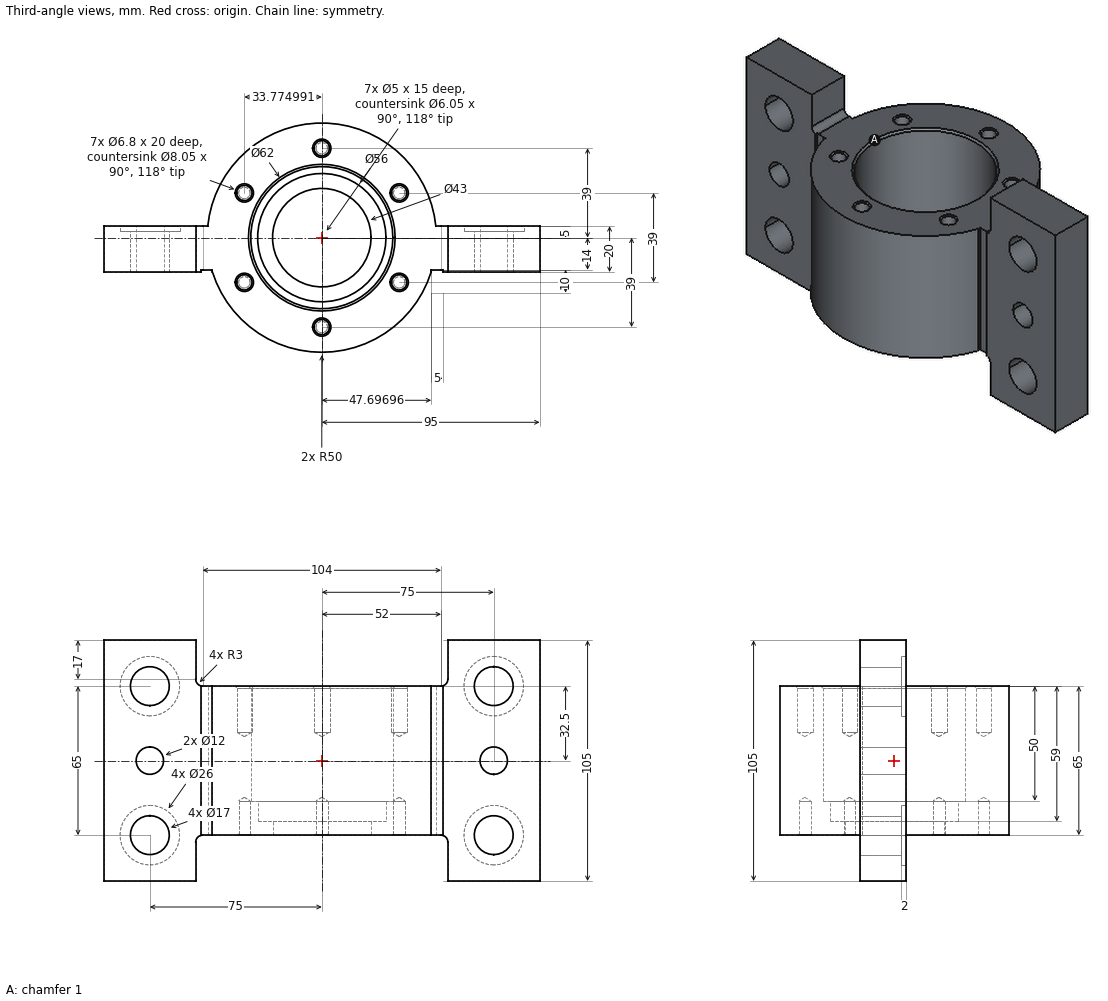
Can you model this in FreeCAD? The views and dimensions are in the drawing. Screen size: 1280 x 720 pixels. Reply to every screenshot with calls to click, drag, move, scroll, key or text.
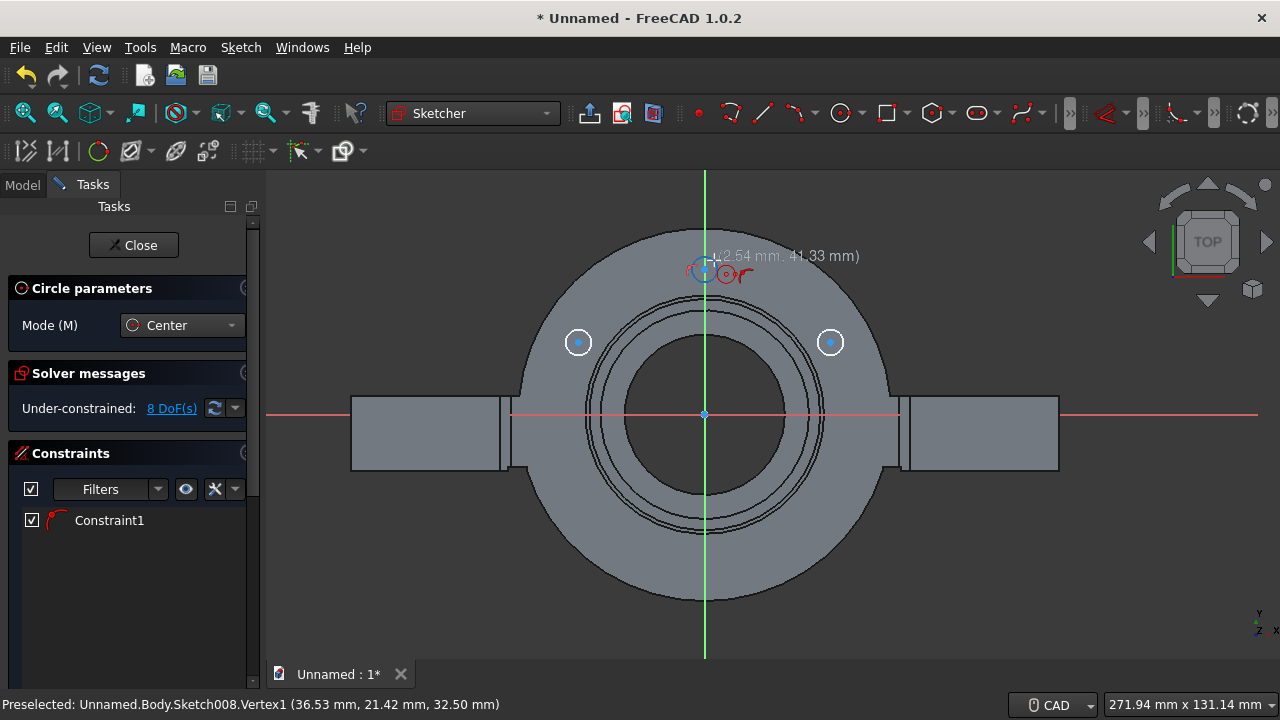
scroll(831, 487, up, 3)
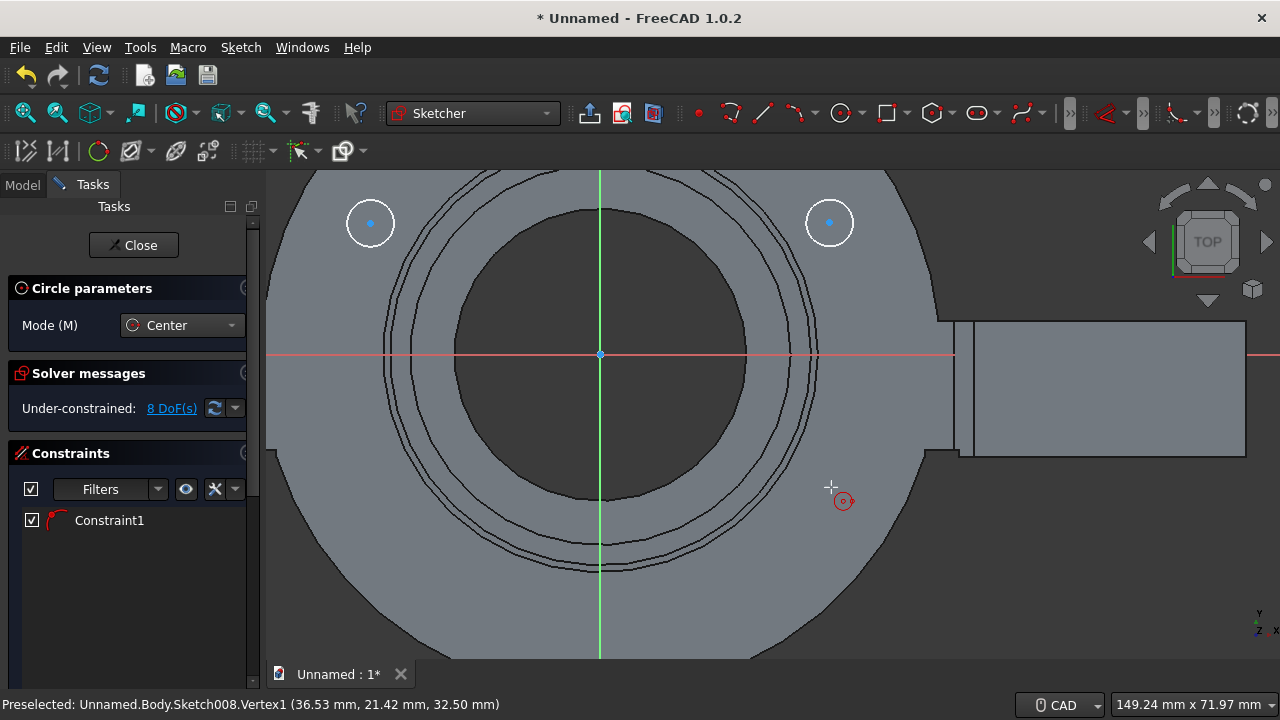
click(830, 487)
click(846, 471)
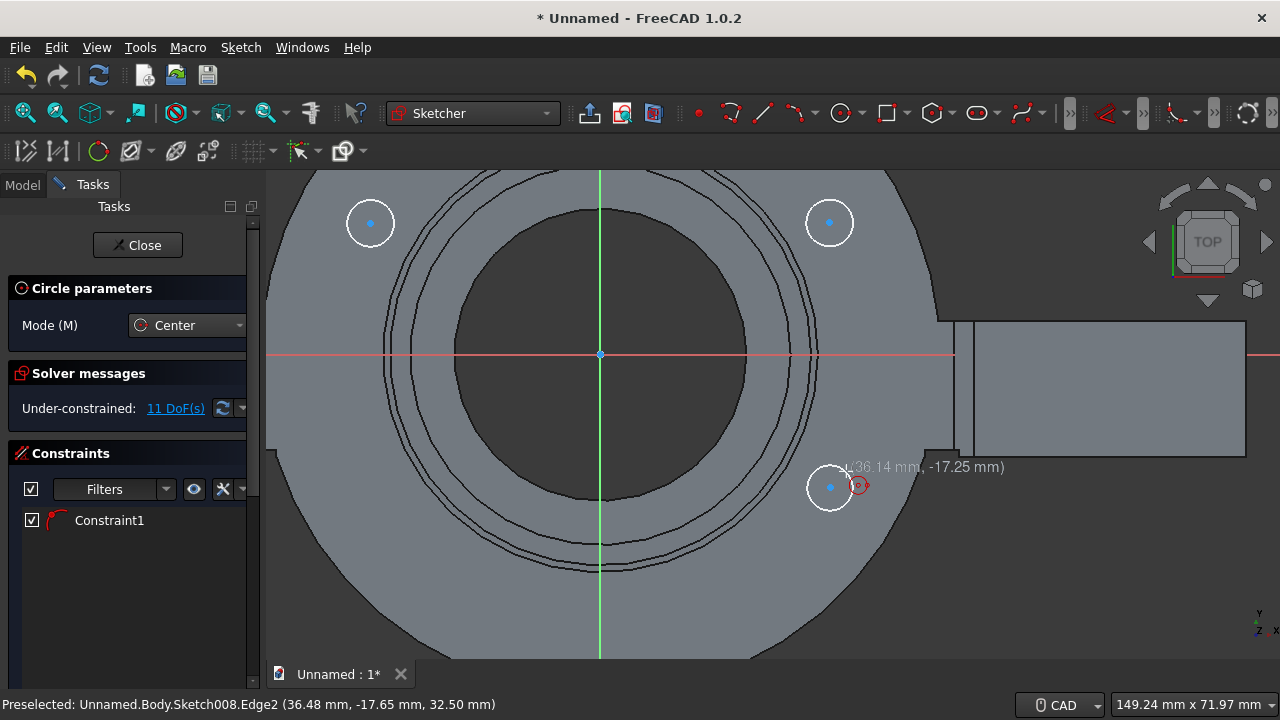
click(600, 620)
click(617, 603)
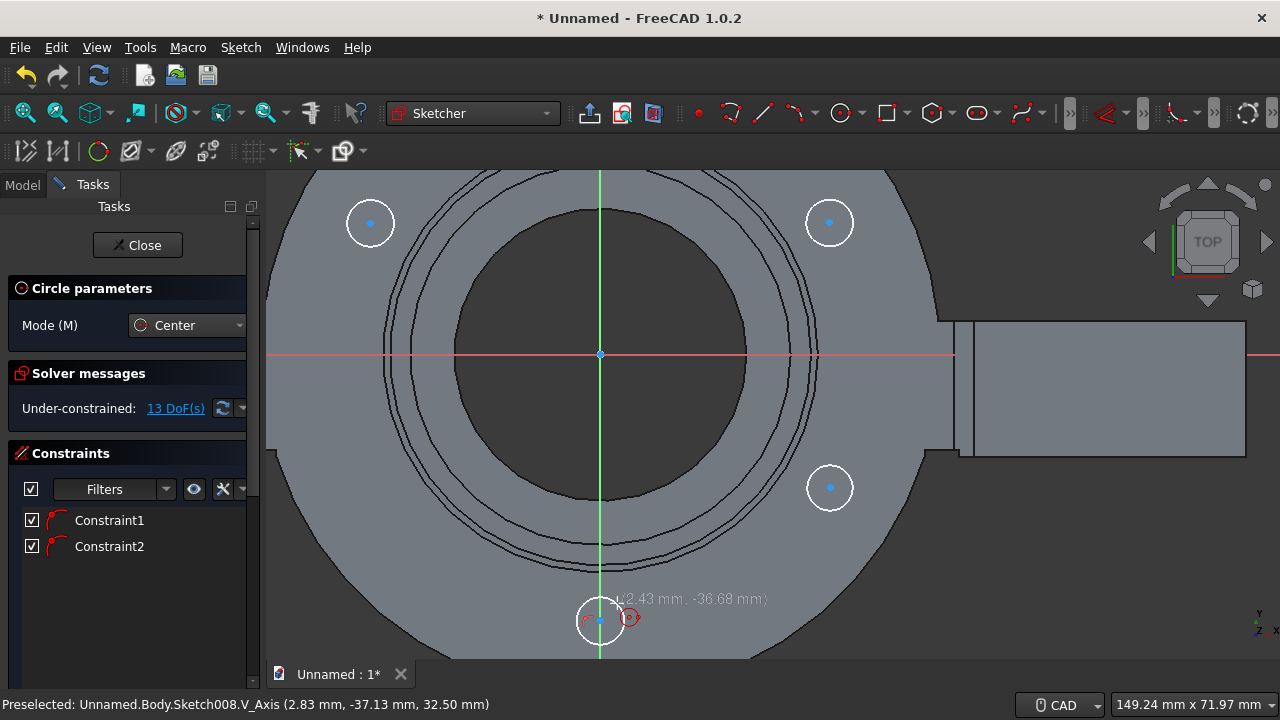
click(371, 487)
click(387, 471)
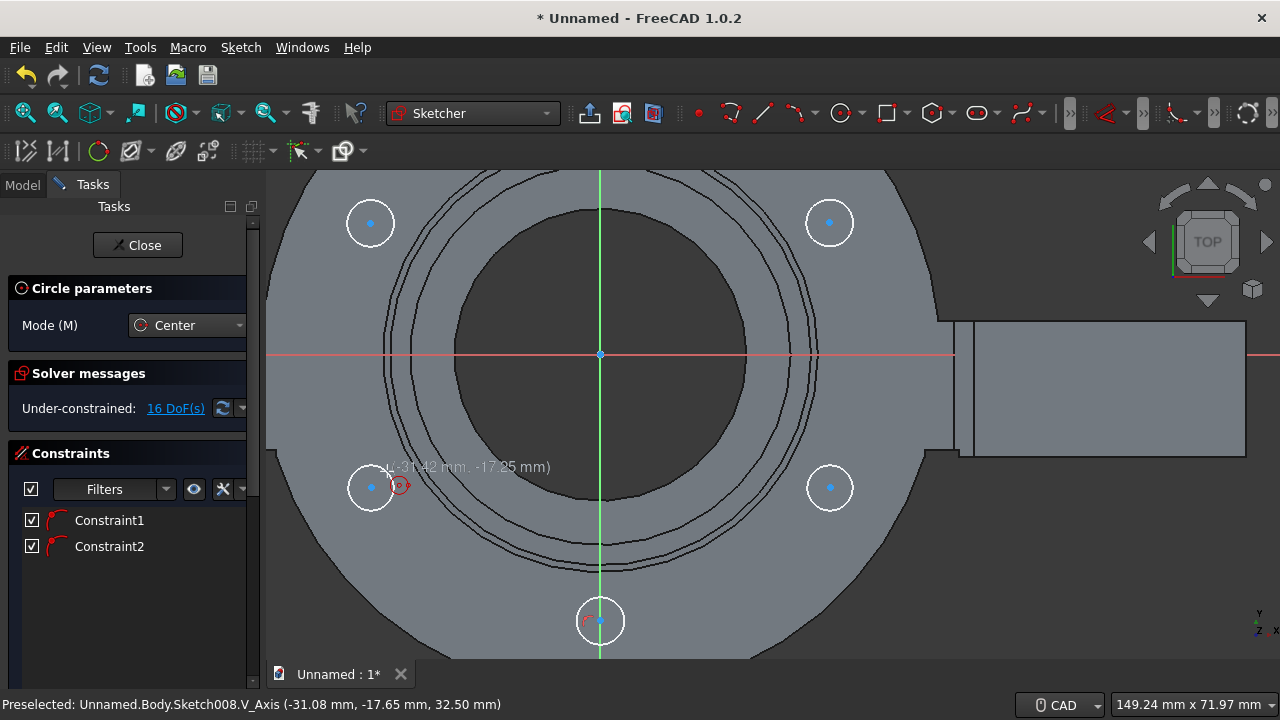
click(600, 355)
click(617, 338)
key(Escape)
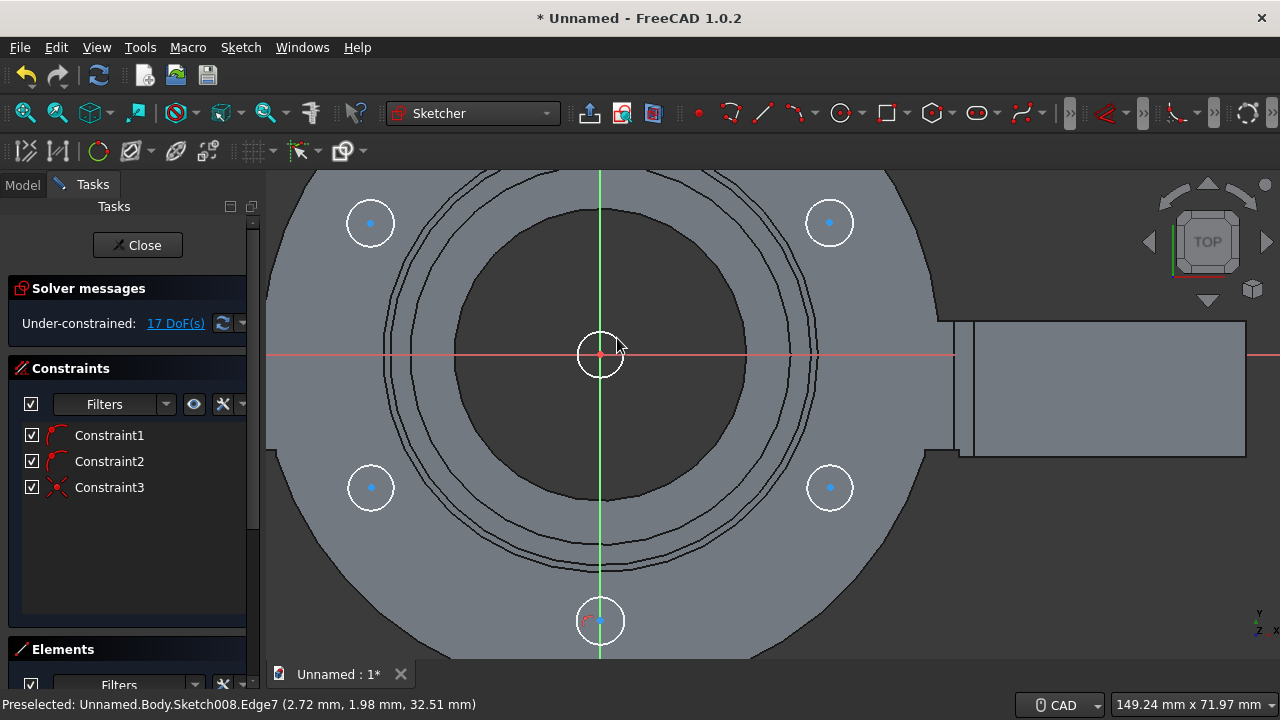
click(387, 207)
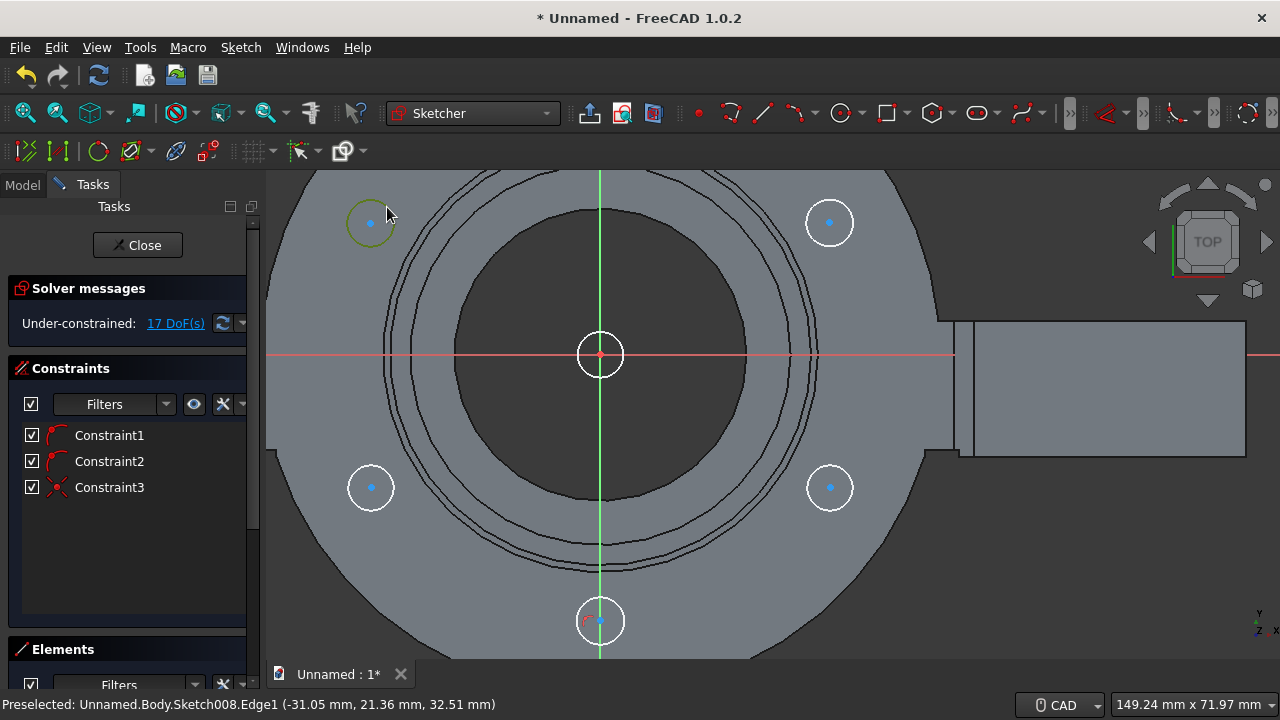
scroll(831, 487, down, 3)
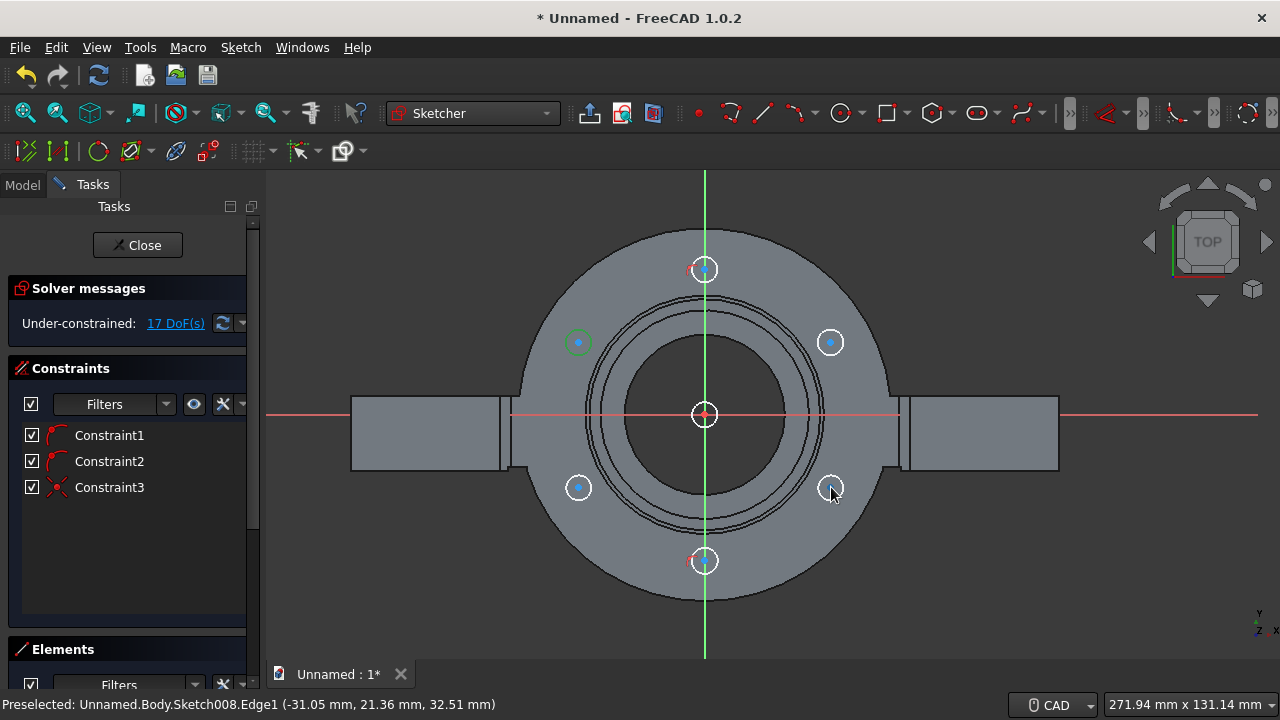
scroll(714, 261, up, 3)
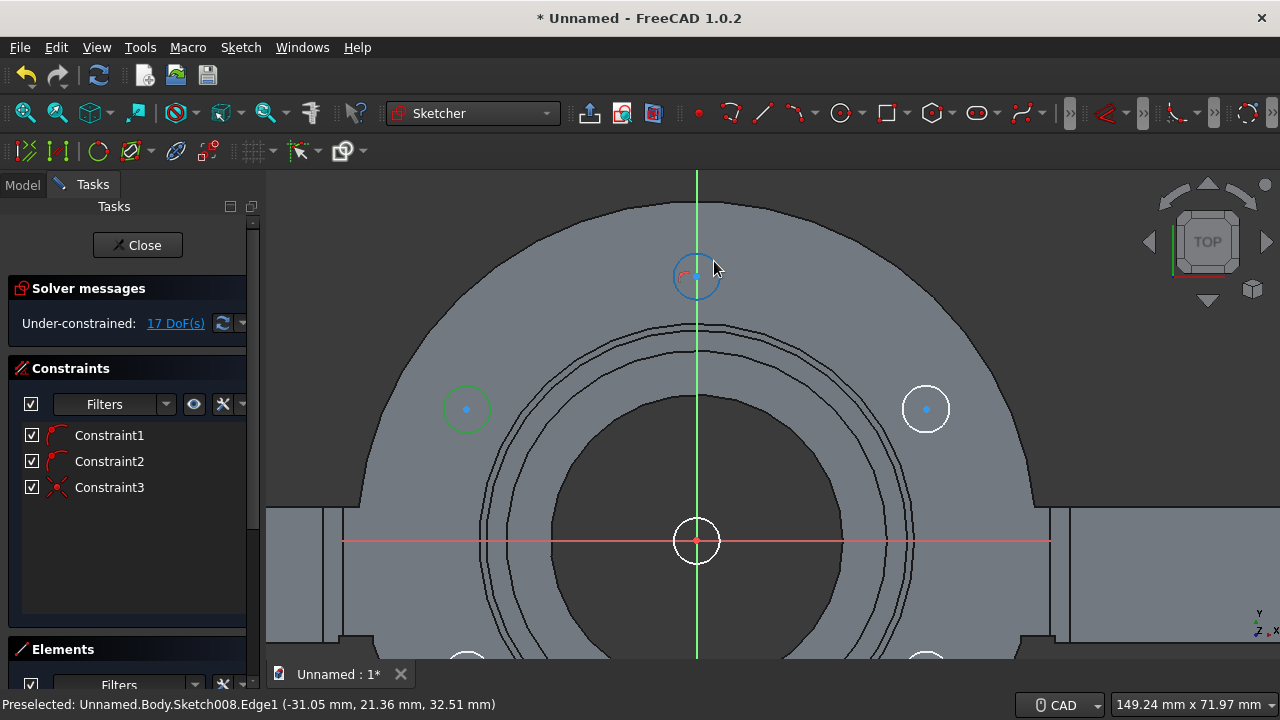
click(713, 260)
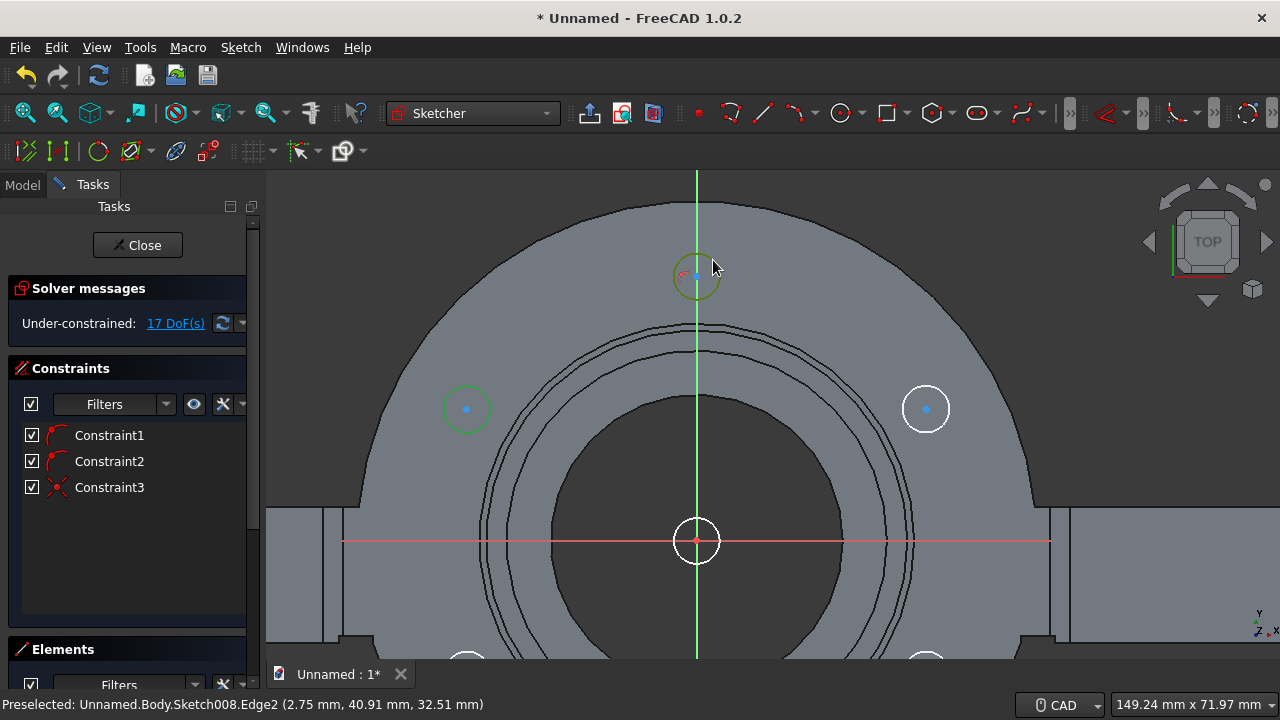
click(942, 393)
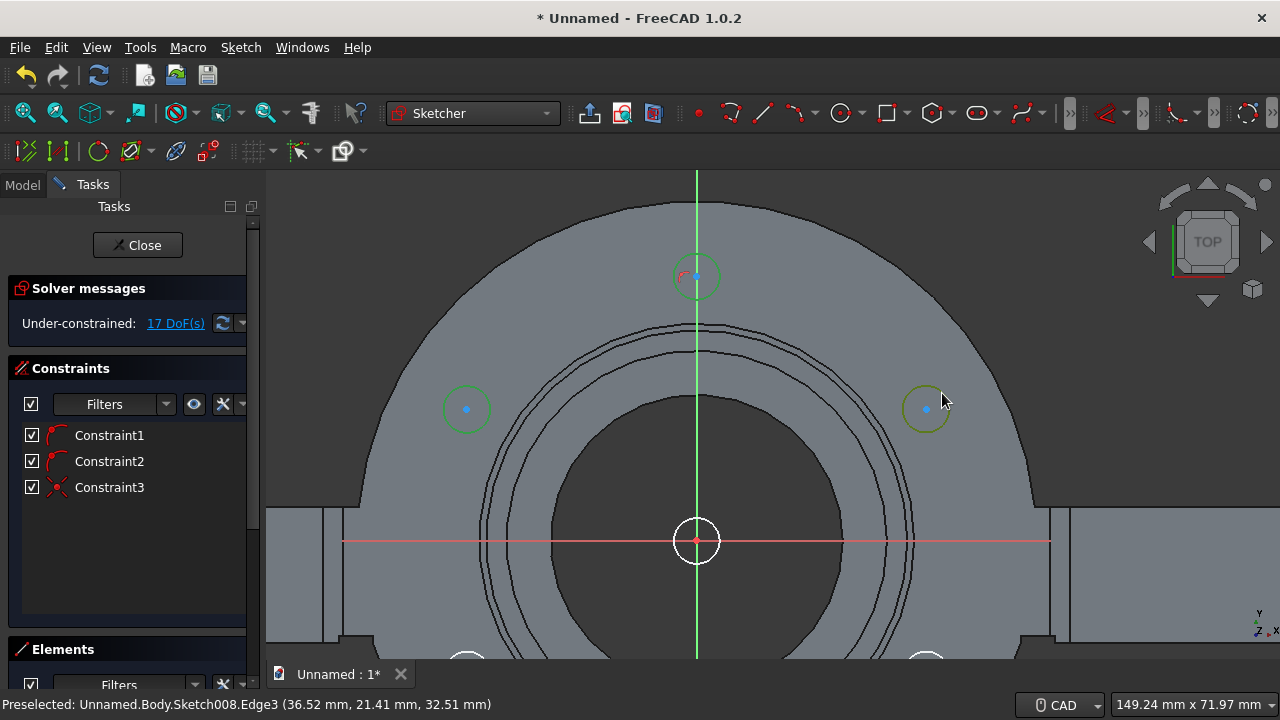
scroll(714, 261, down, 3)